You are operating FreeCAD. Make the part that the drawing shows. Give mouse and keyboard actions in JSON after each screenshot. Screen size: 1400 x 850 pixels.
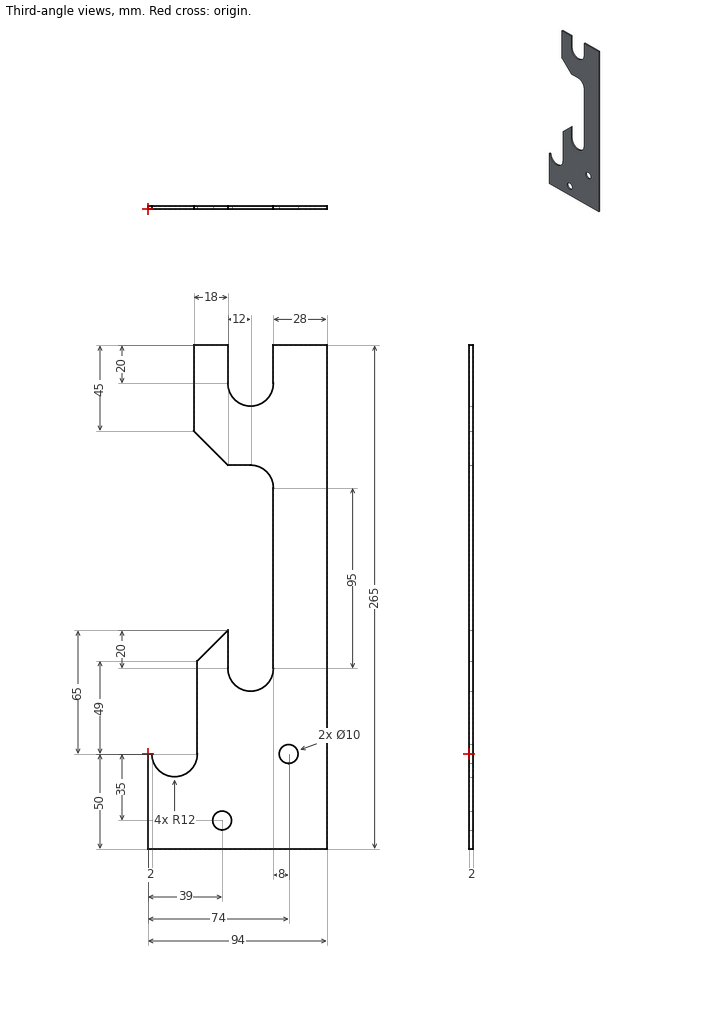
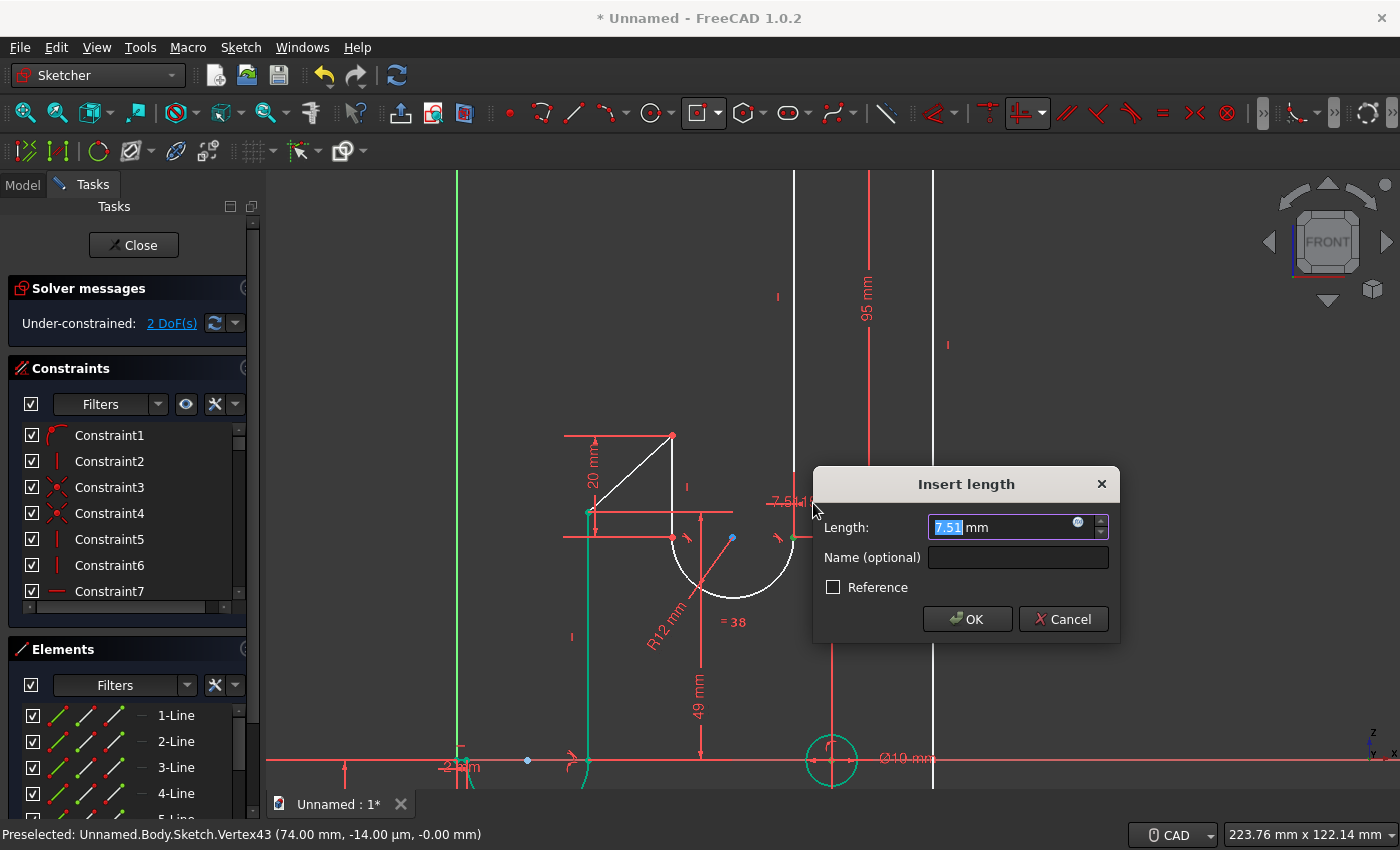
{"action": "type", "text": "8"}
{"action": "key", "text": "Return"}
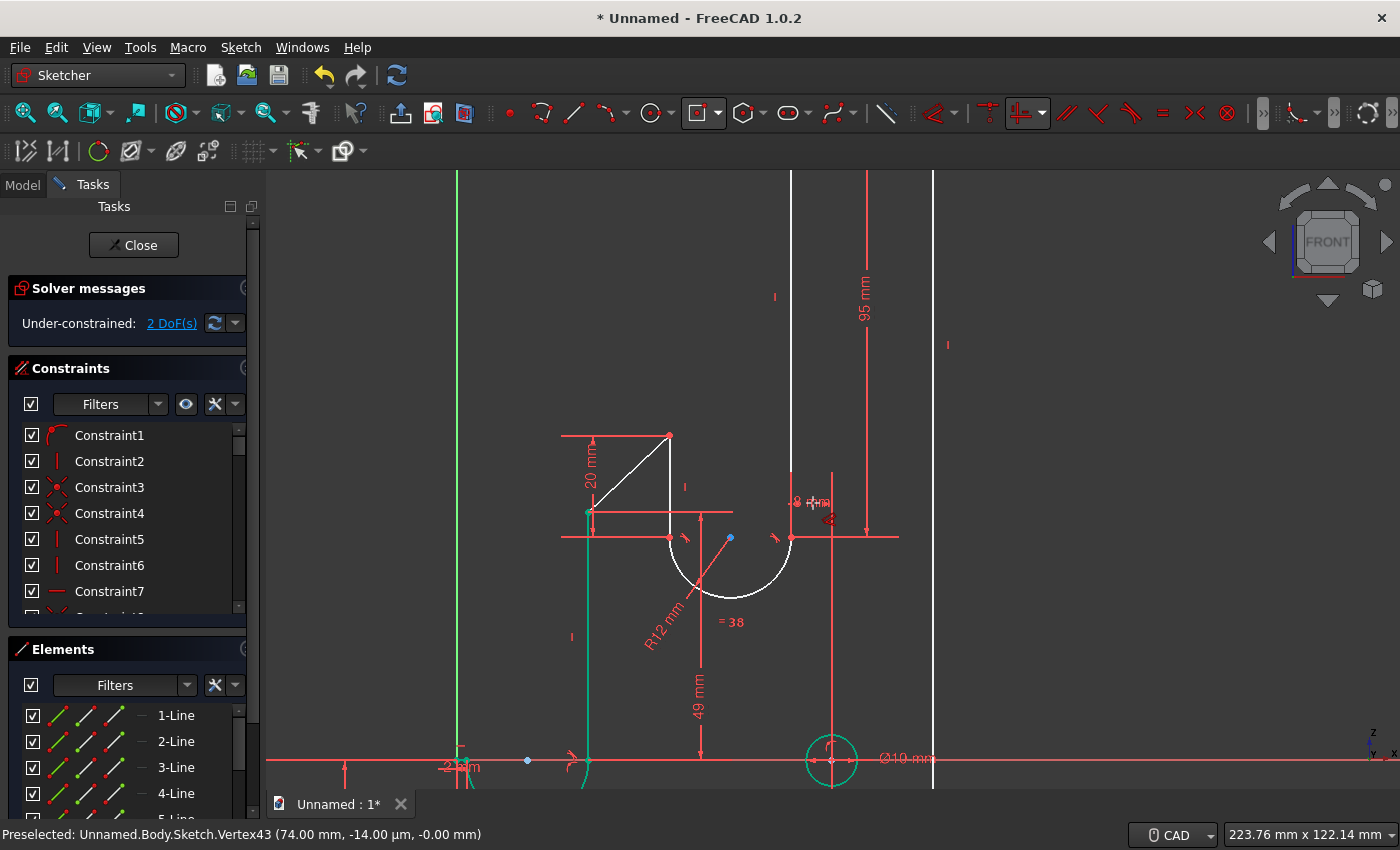
{"action": "left_click", "coordinate": [933, 612]}
{"action": "left_click", "coordinate": [967, 480]}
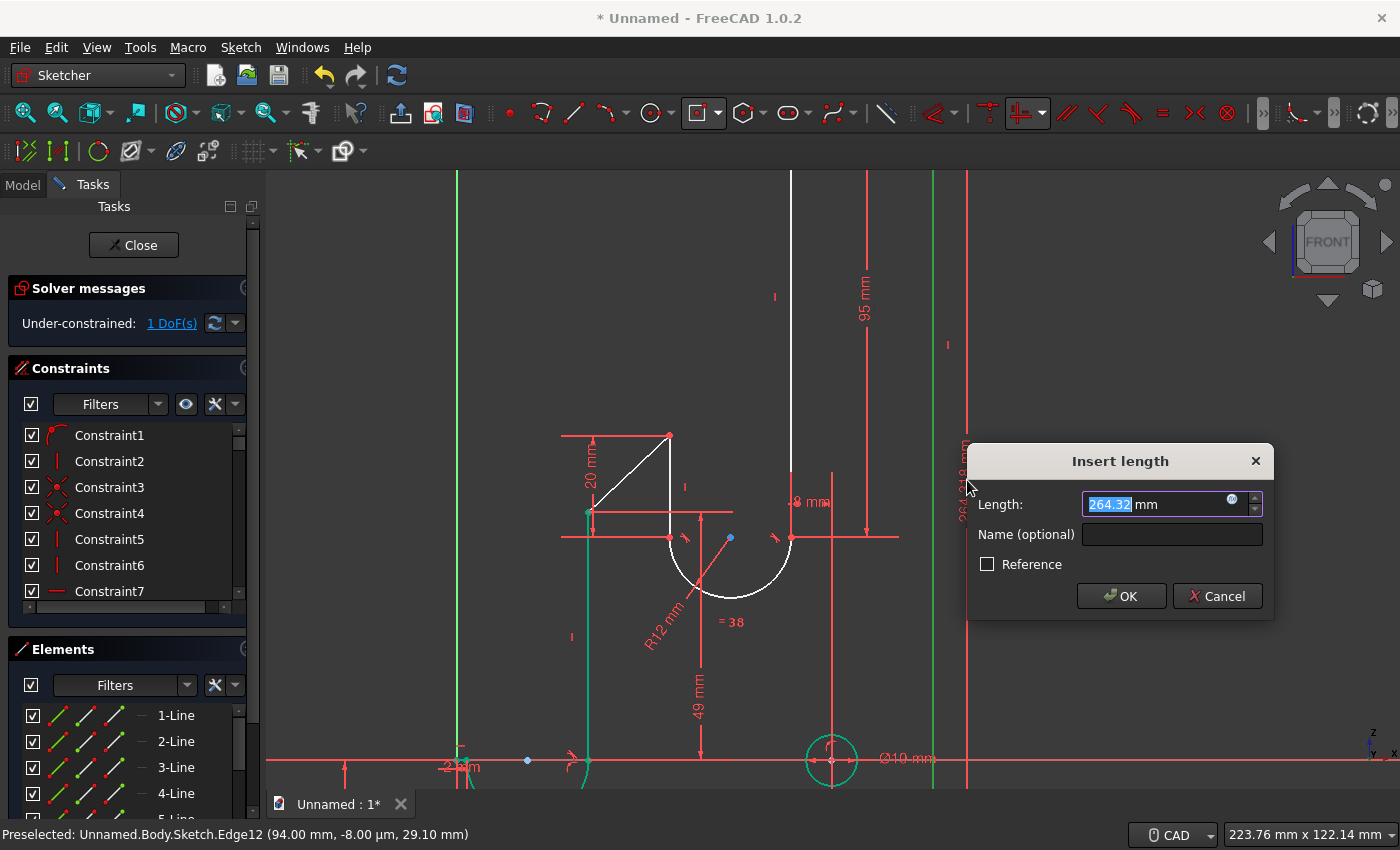
{"action": "type", "text": "265"}
{"action": "key", "text": "Return"}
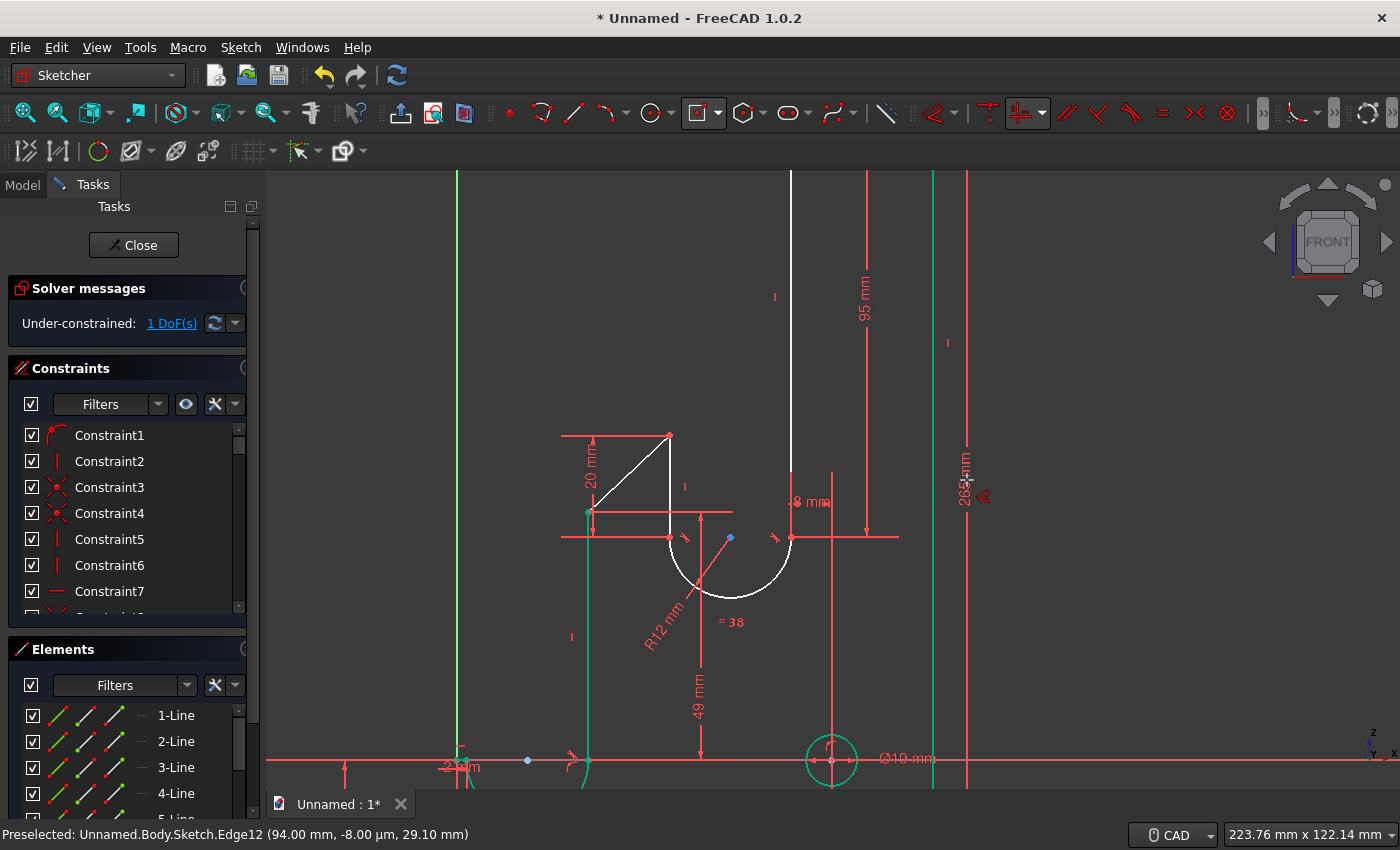
{"action": "left_click", "coordinate": [670, 436]}
{"action": "left_click", "coordinate": [423, 598]}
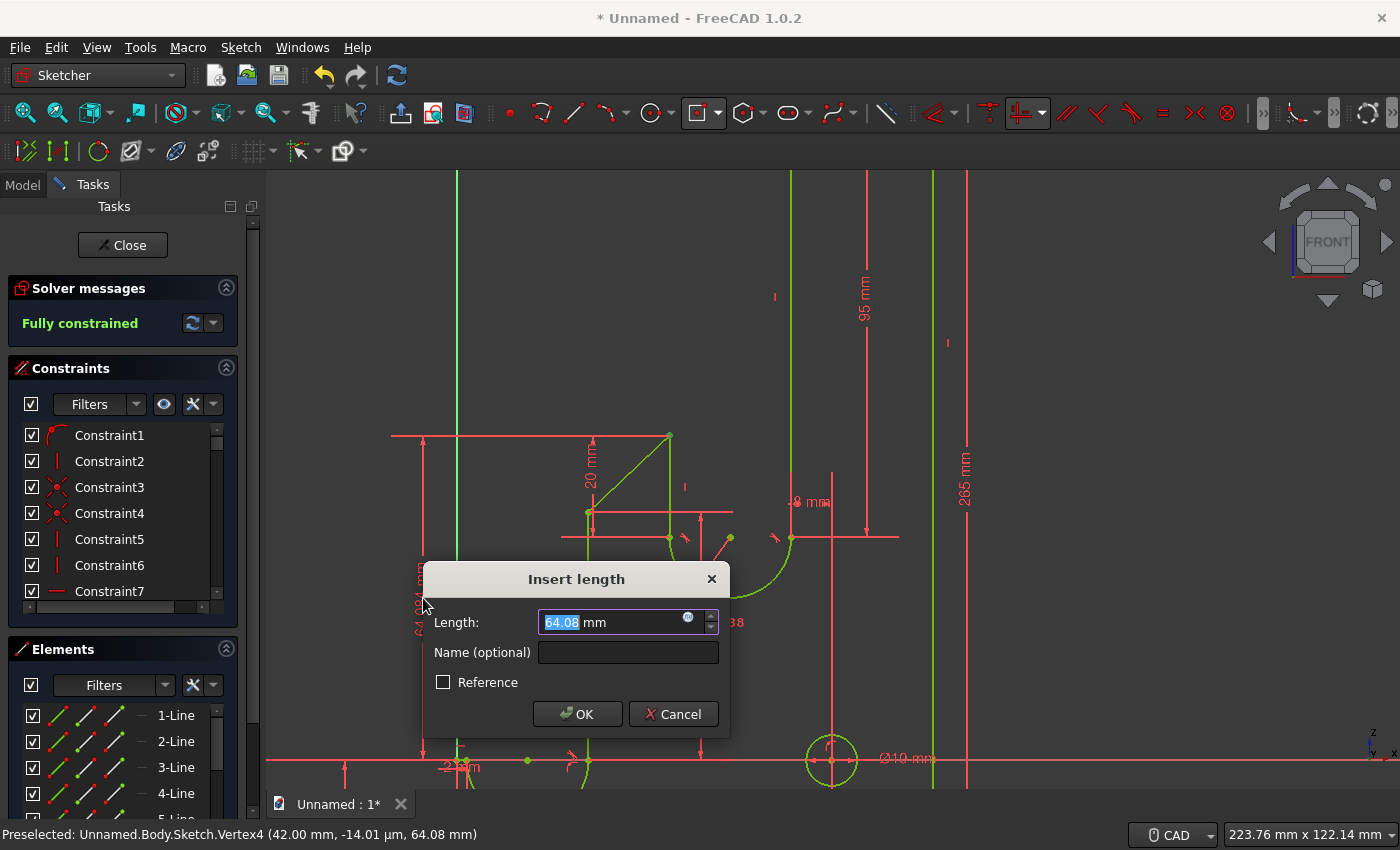
{"action": "type", "text": "65"}
{"action": "key", "text": "Return"}
{"action": "key", "text": "Escape"}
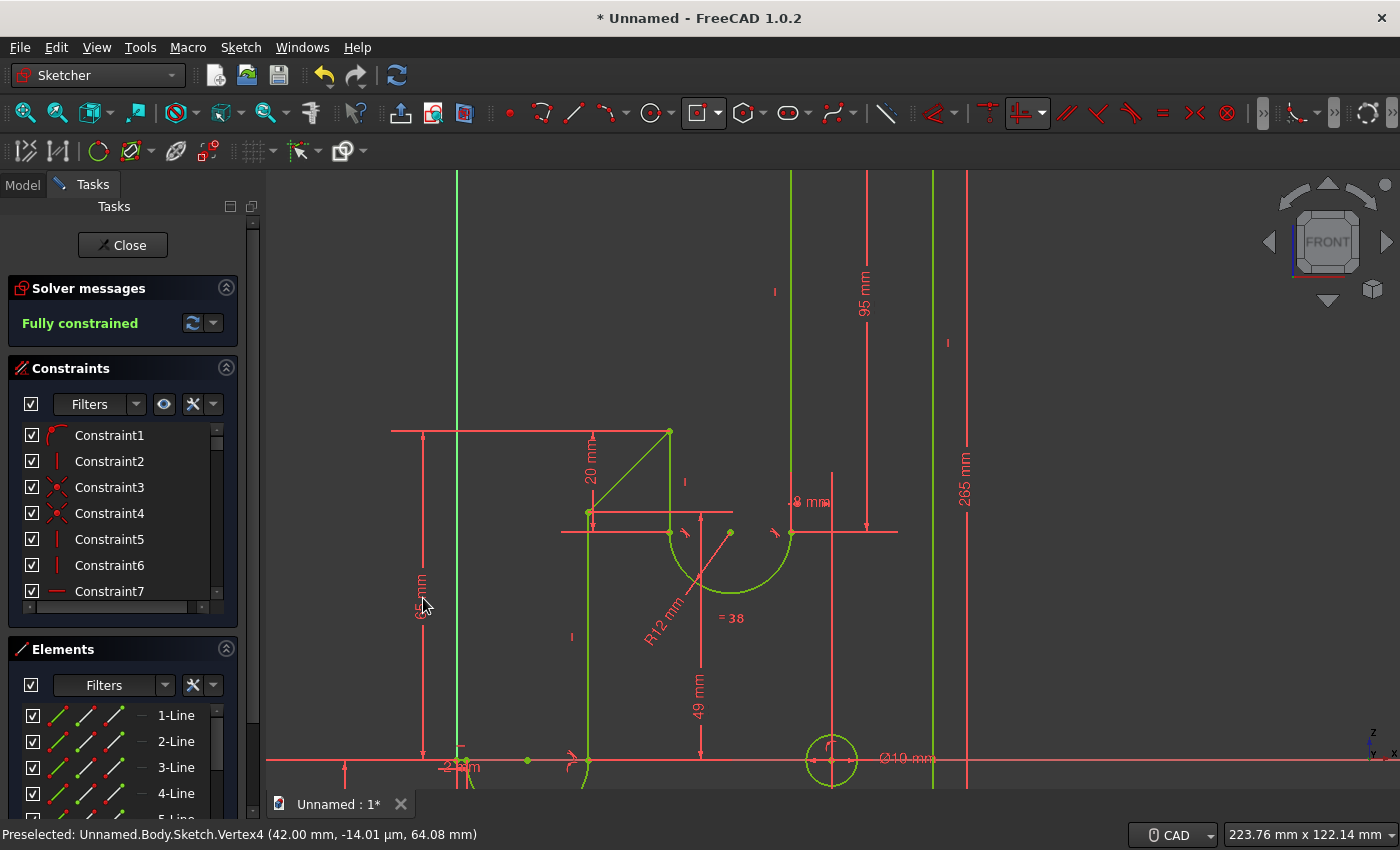
{"action": "left_click", "coordinate": [123, 245]}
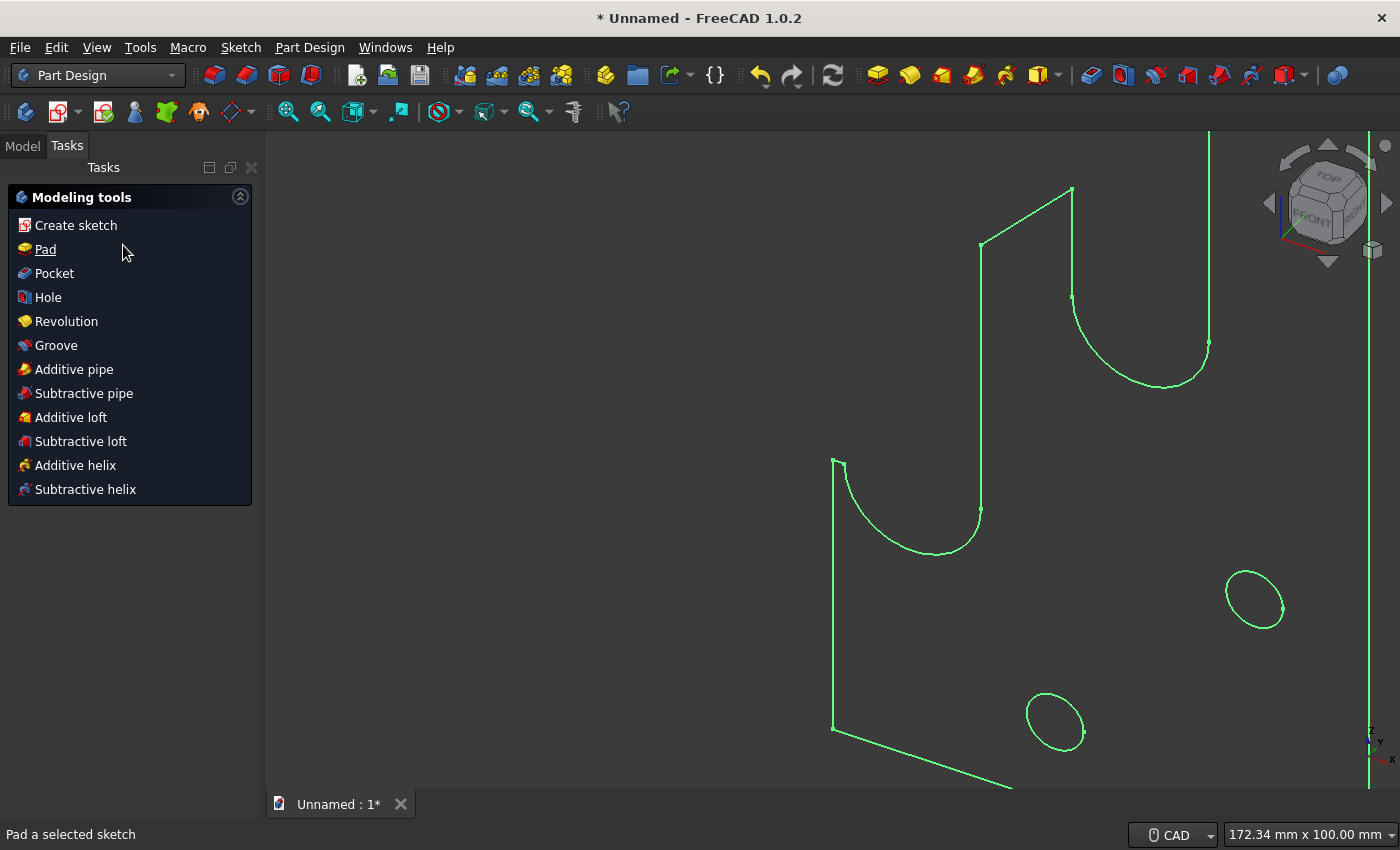
{"action": "left_click", "coordinate": [878, 76]}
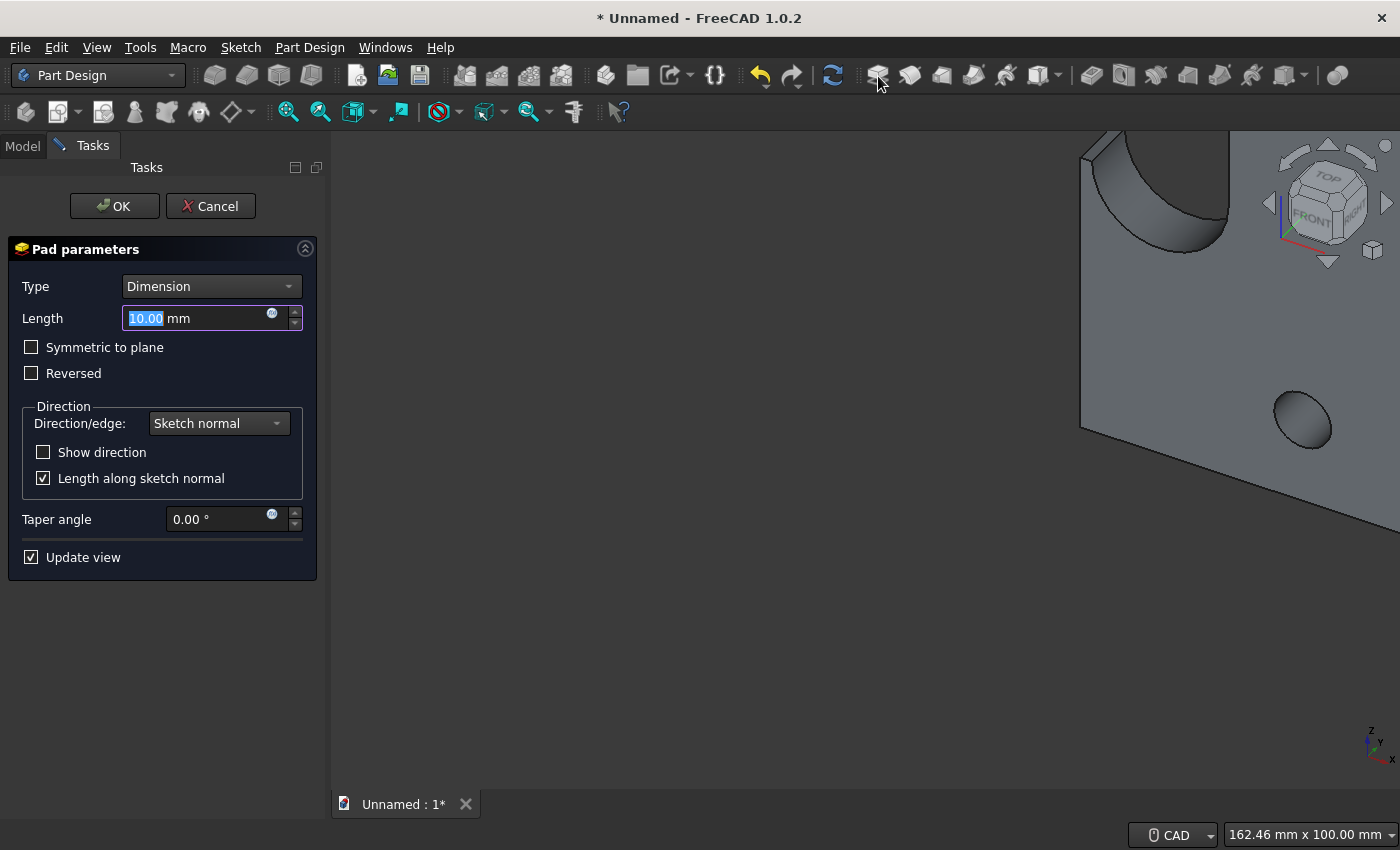
{"action": "type", "text": "2"}
{"action": "key", "text": "Tab"}